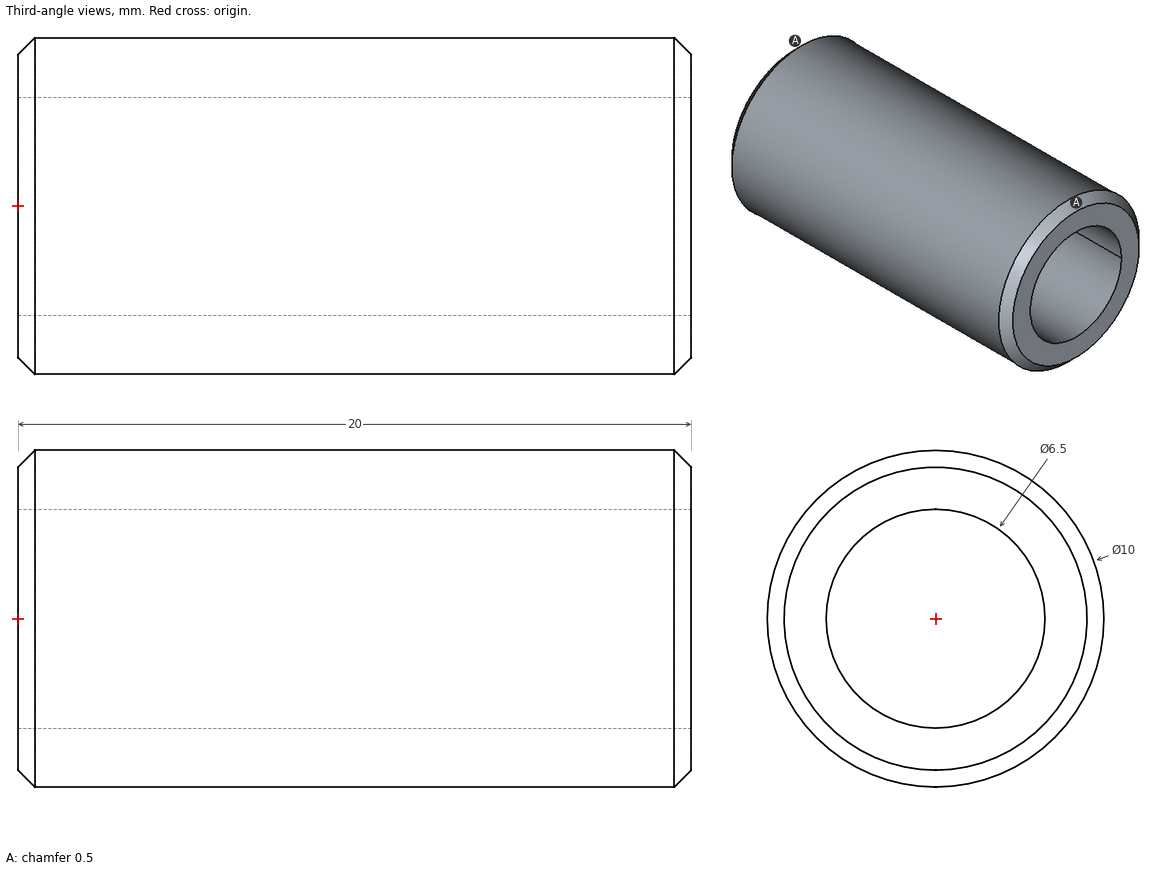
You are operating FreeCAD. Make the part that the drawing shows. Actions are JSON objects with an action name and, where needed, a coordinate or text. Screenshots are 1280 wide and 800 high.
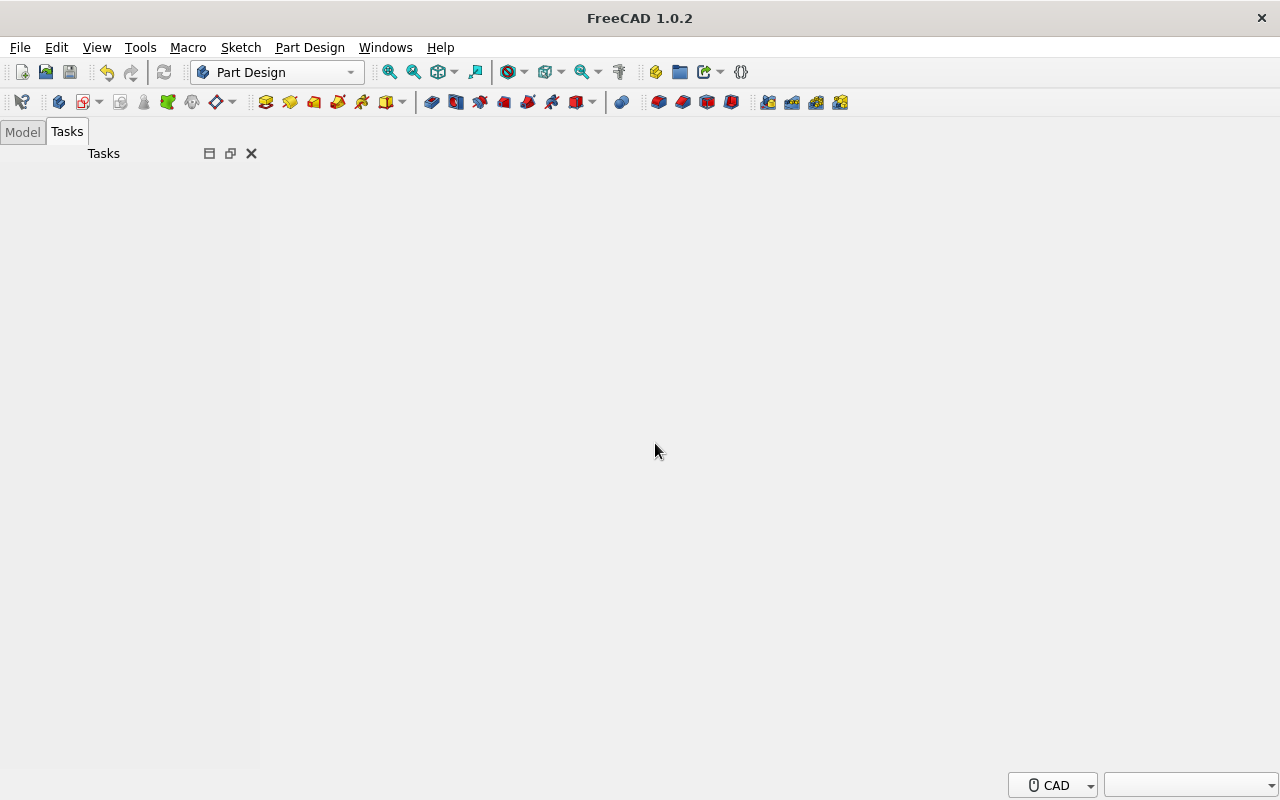
{"action": "left_click", "coordinate": [22, 72]}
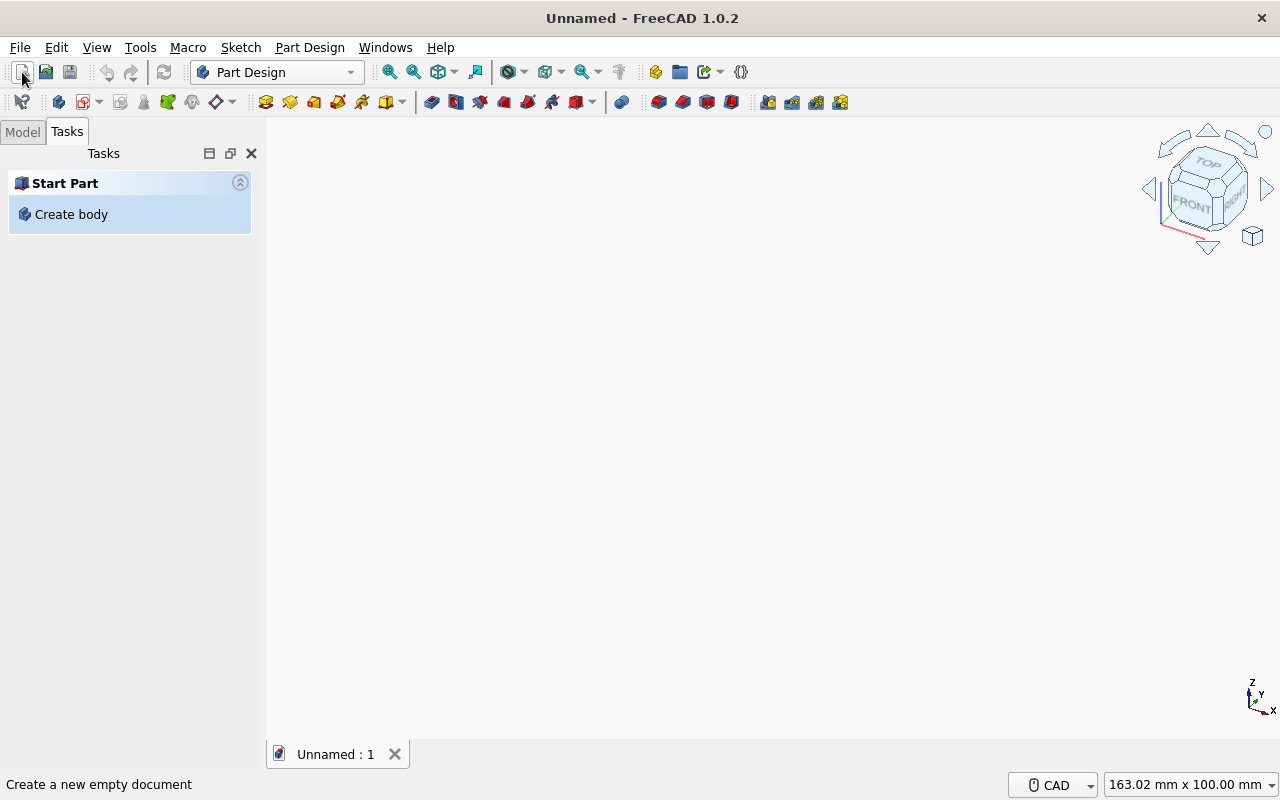
{"action": "left_click", "coordinate": [84, 102]}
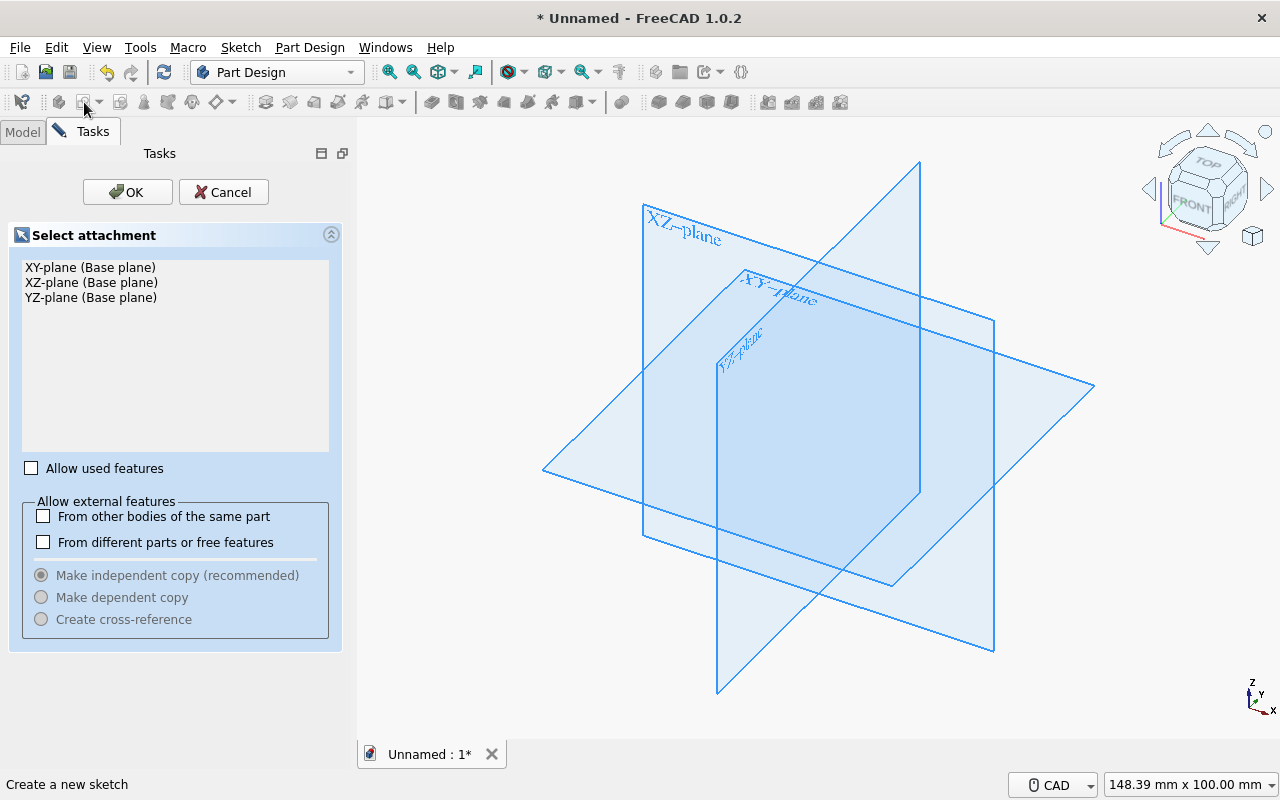
{"action": "left_click", "coordinate": [82, 298]}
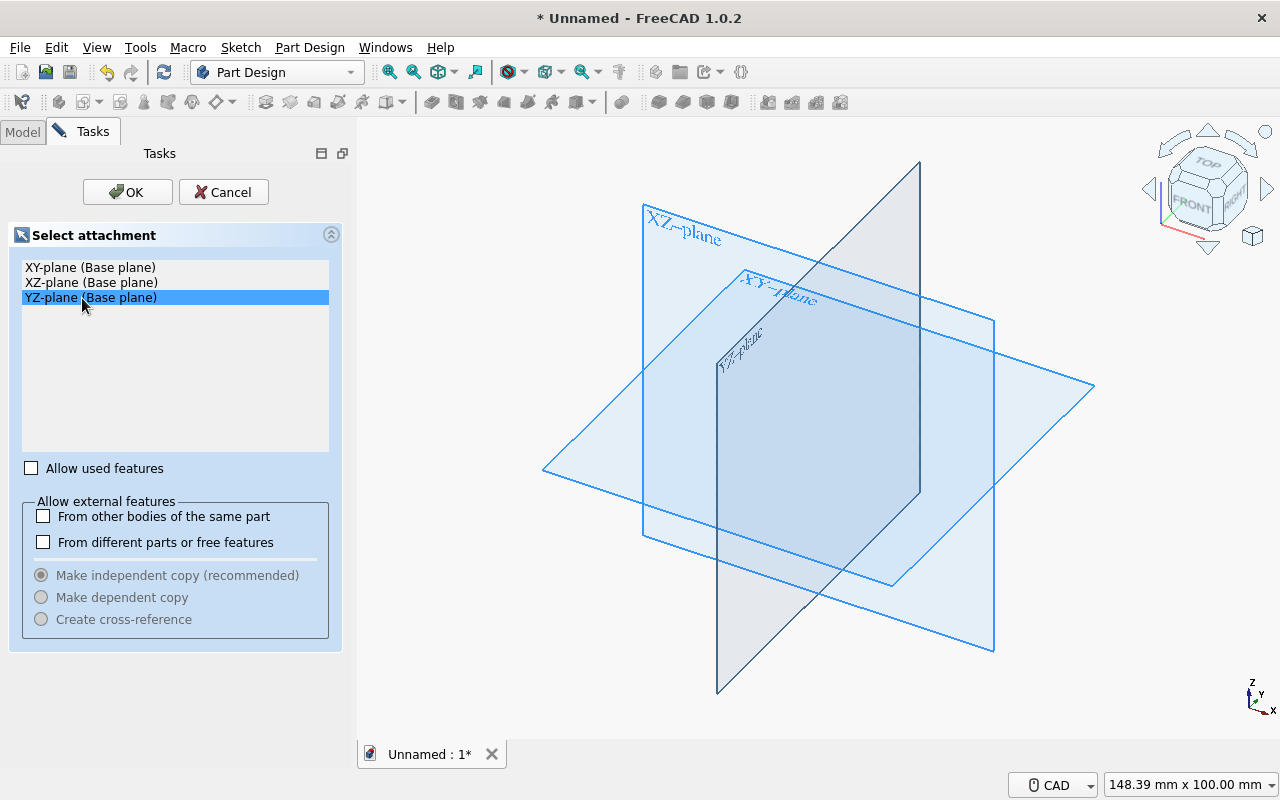
{"action": "left_click", "coordinate": [128, 192]}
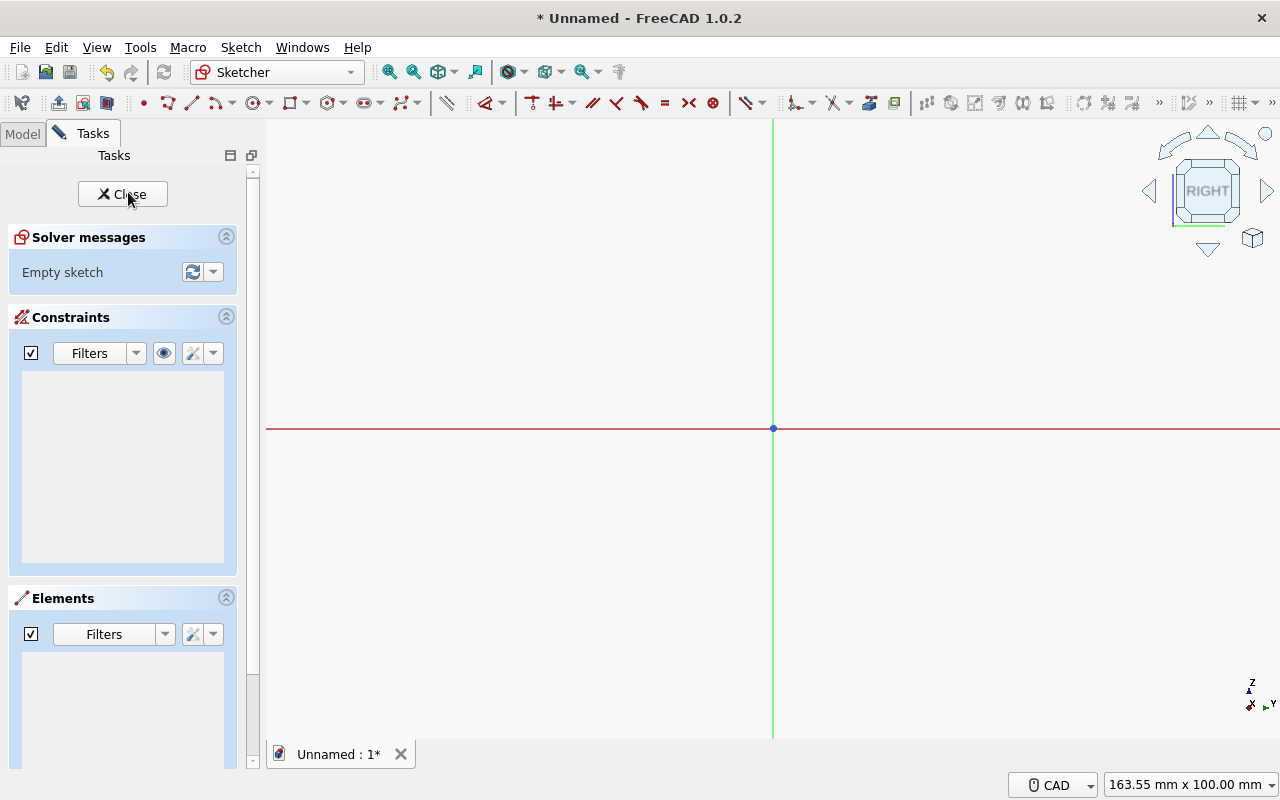
{"action": "scroll", "coordinate": [787, 429], "scroll_direction": "up", "scroll_amount": 9}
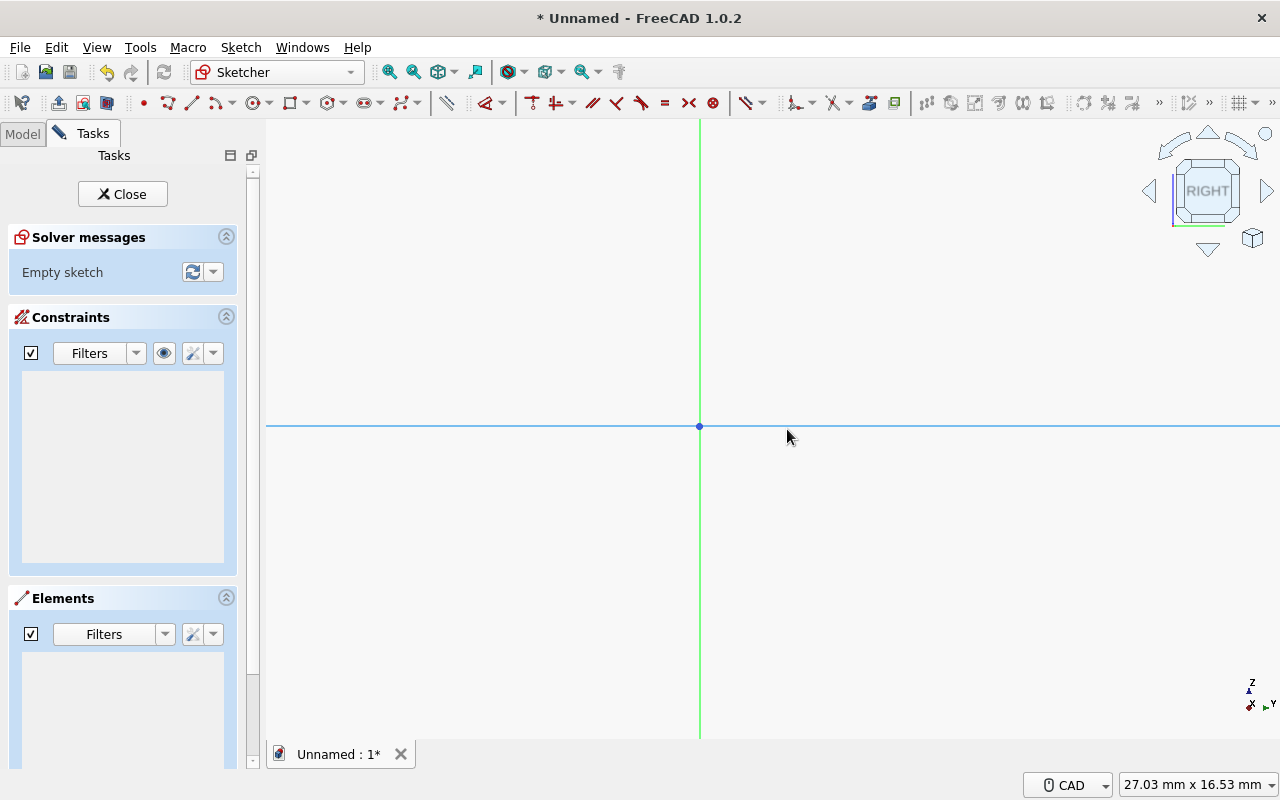
{"action": "left_click", "coordinate": [254, 104]}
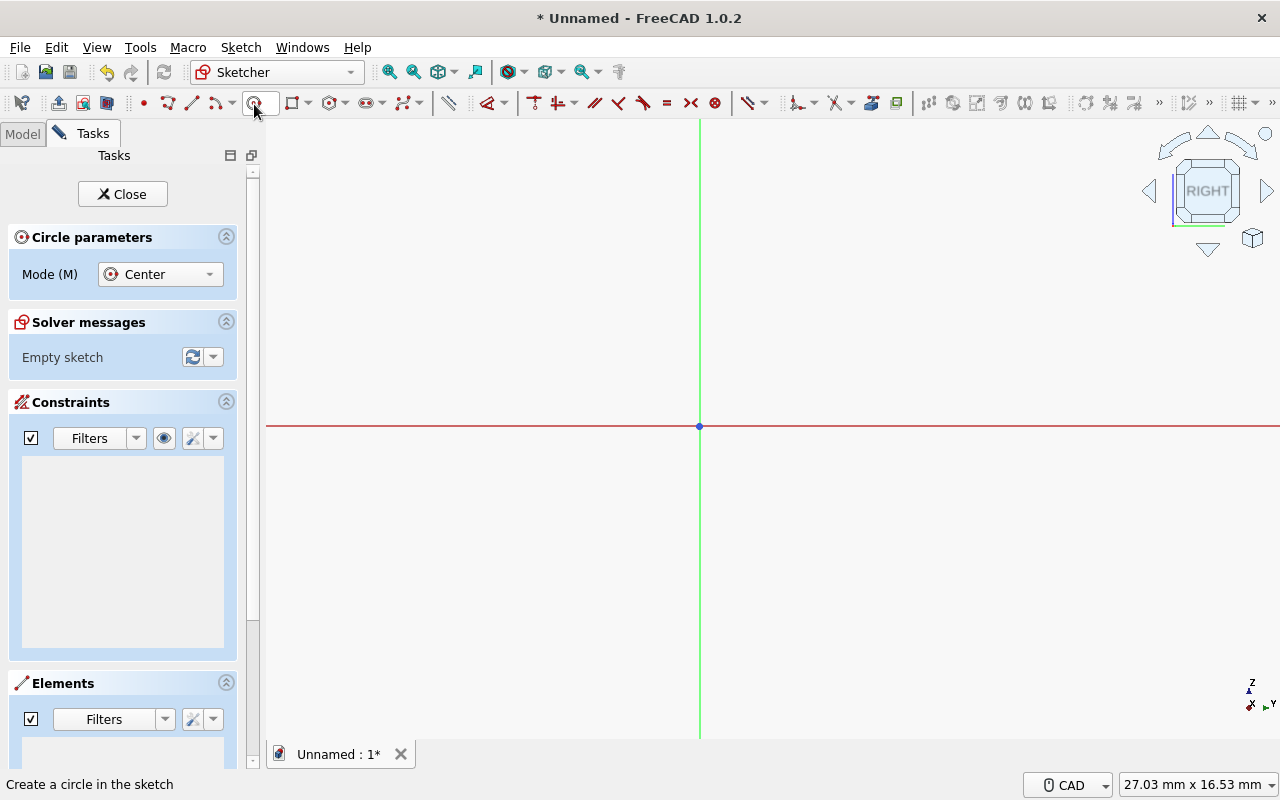
{"action": "left_click", "coordinate": [700, 426]}
{"action": "left_click", "coordinate": [832, 294]}
{"action": "key", "text": "Escape"}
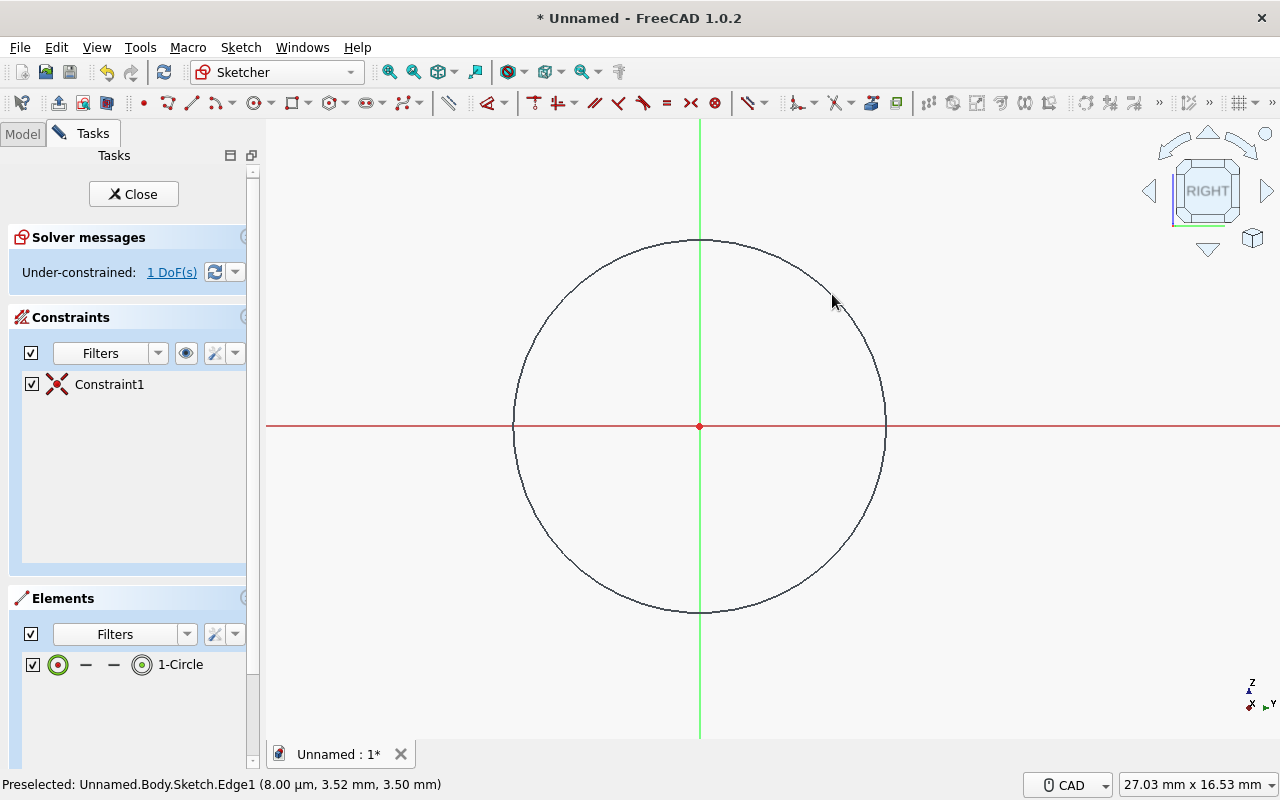
{"action": "key", "text": "d"}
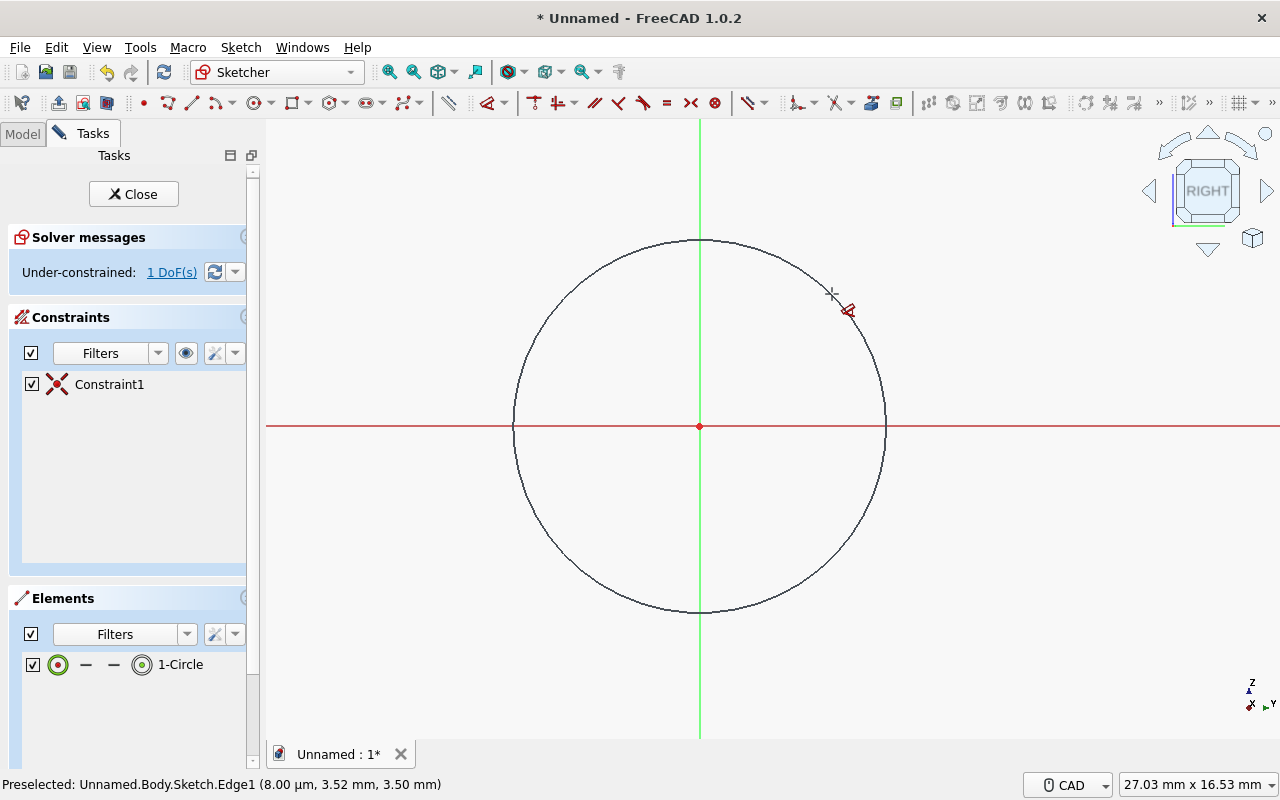
{"action": "left_click", "coordinate": [831, 294]}
{"action": "left_click", "coordinate": [854, 271]}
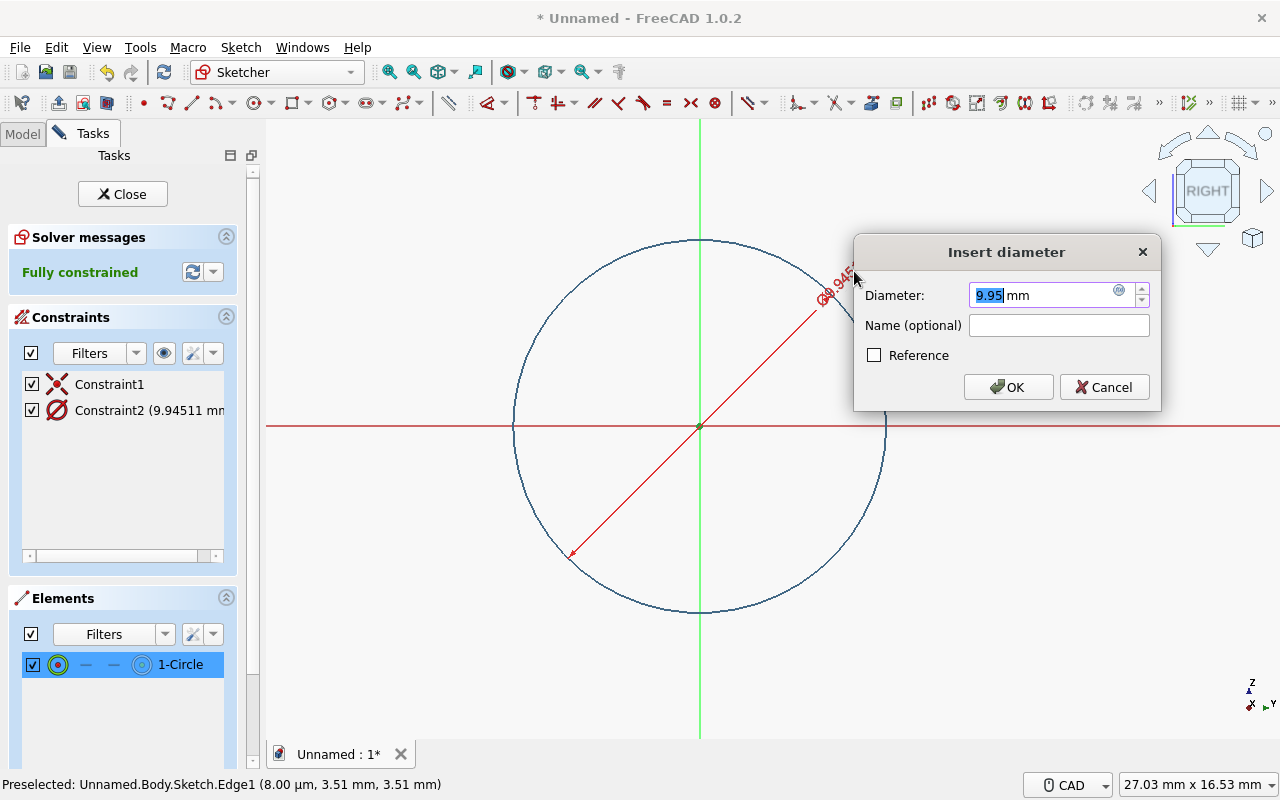
{"action": "type", "text": "10"}
{"action": "key", "text": "Return"}
{"action": "key", "text": "Escape"}